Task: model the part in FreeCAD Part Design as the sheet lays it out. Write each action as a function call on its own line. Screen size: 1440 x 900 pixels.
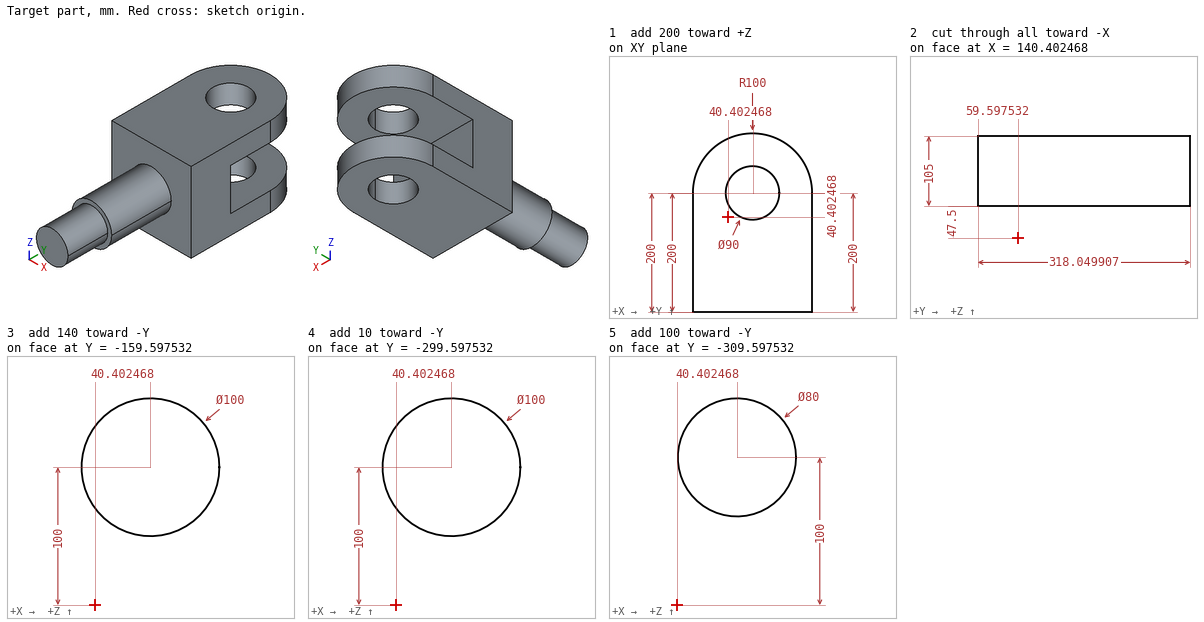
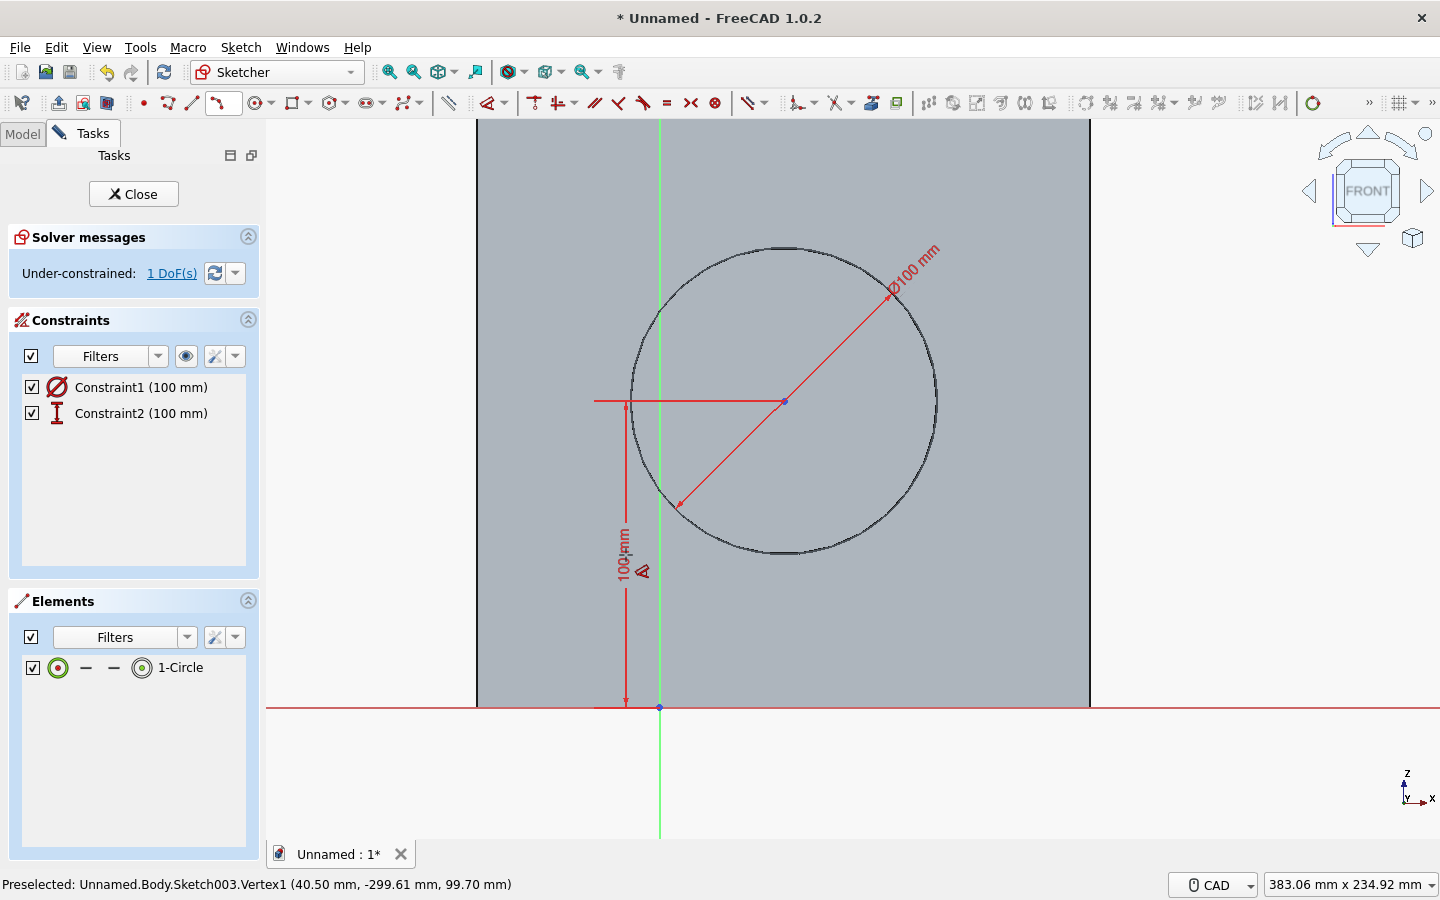
click(784, 401)
click(722, 742)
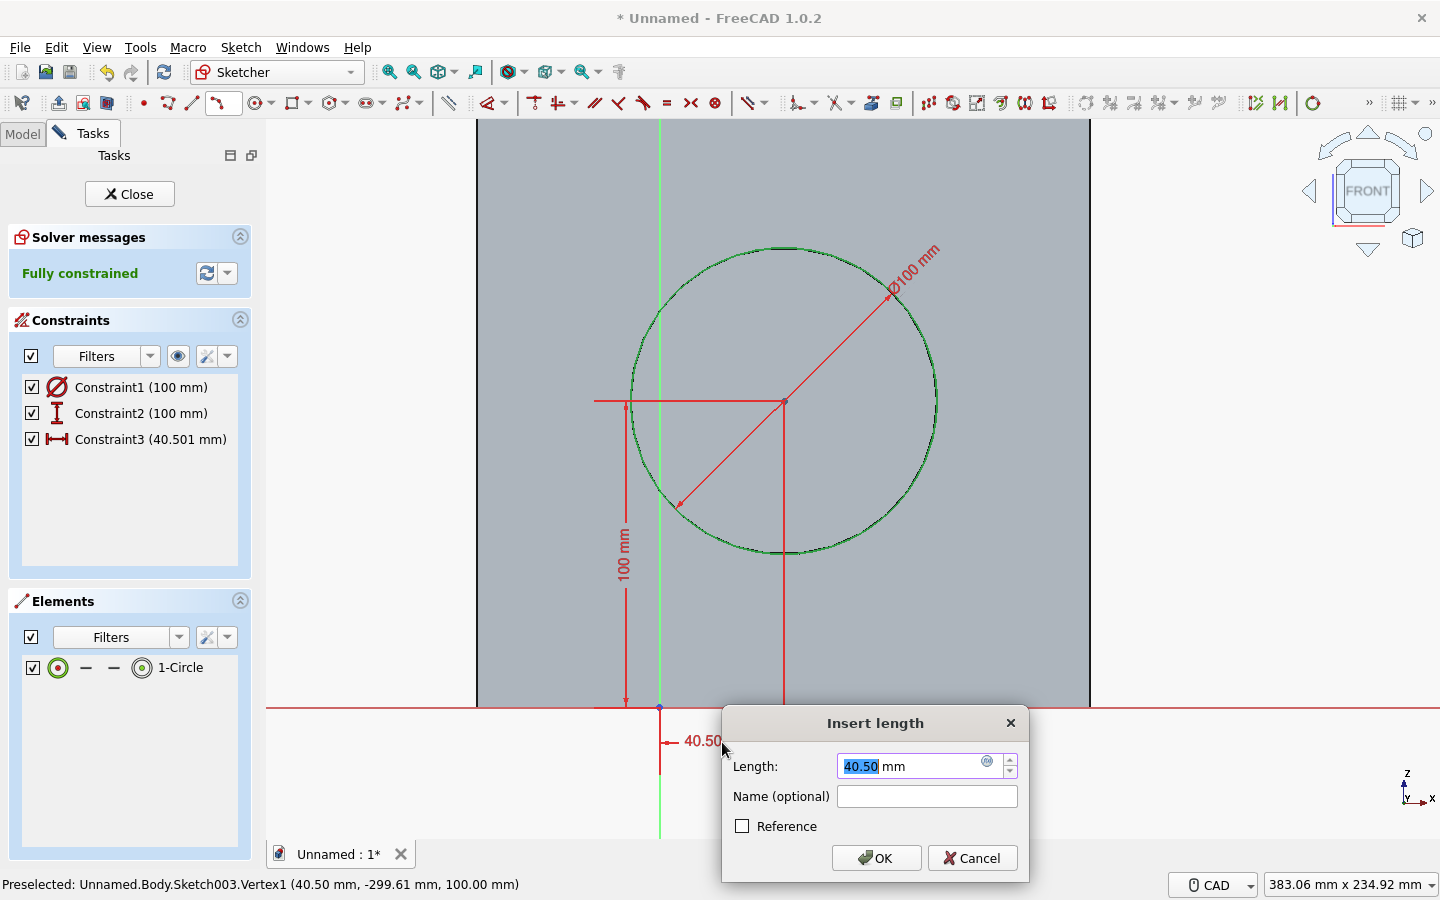
text(40.402468)
key(Return)
key(Escape)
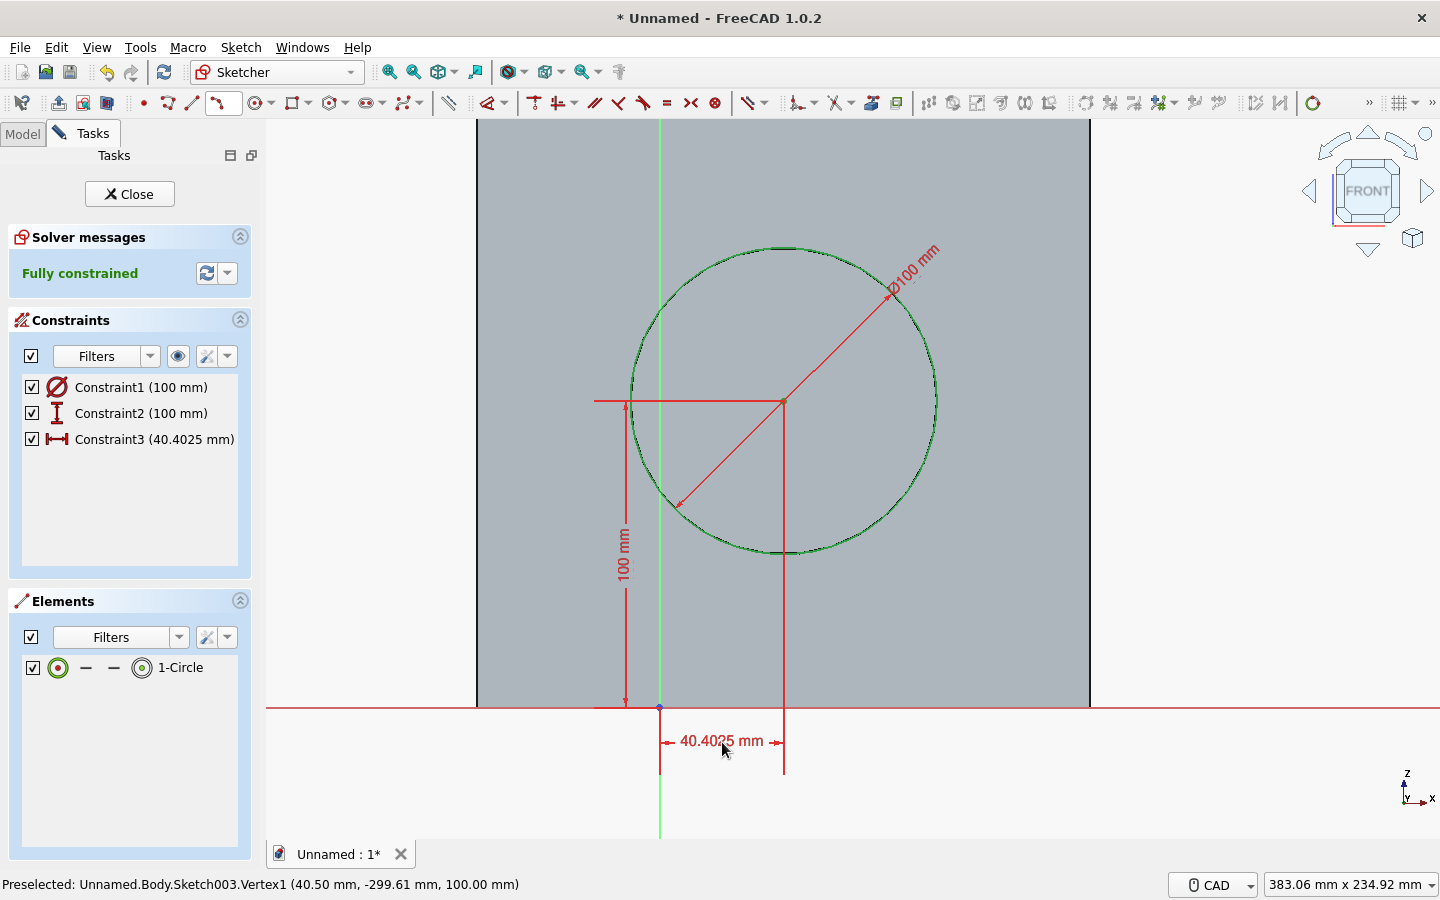
click(130, 194)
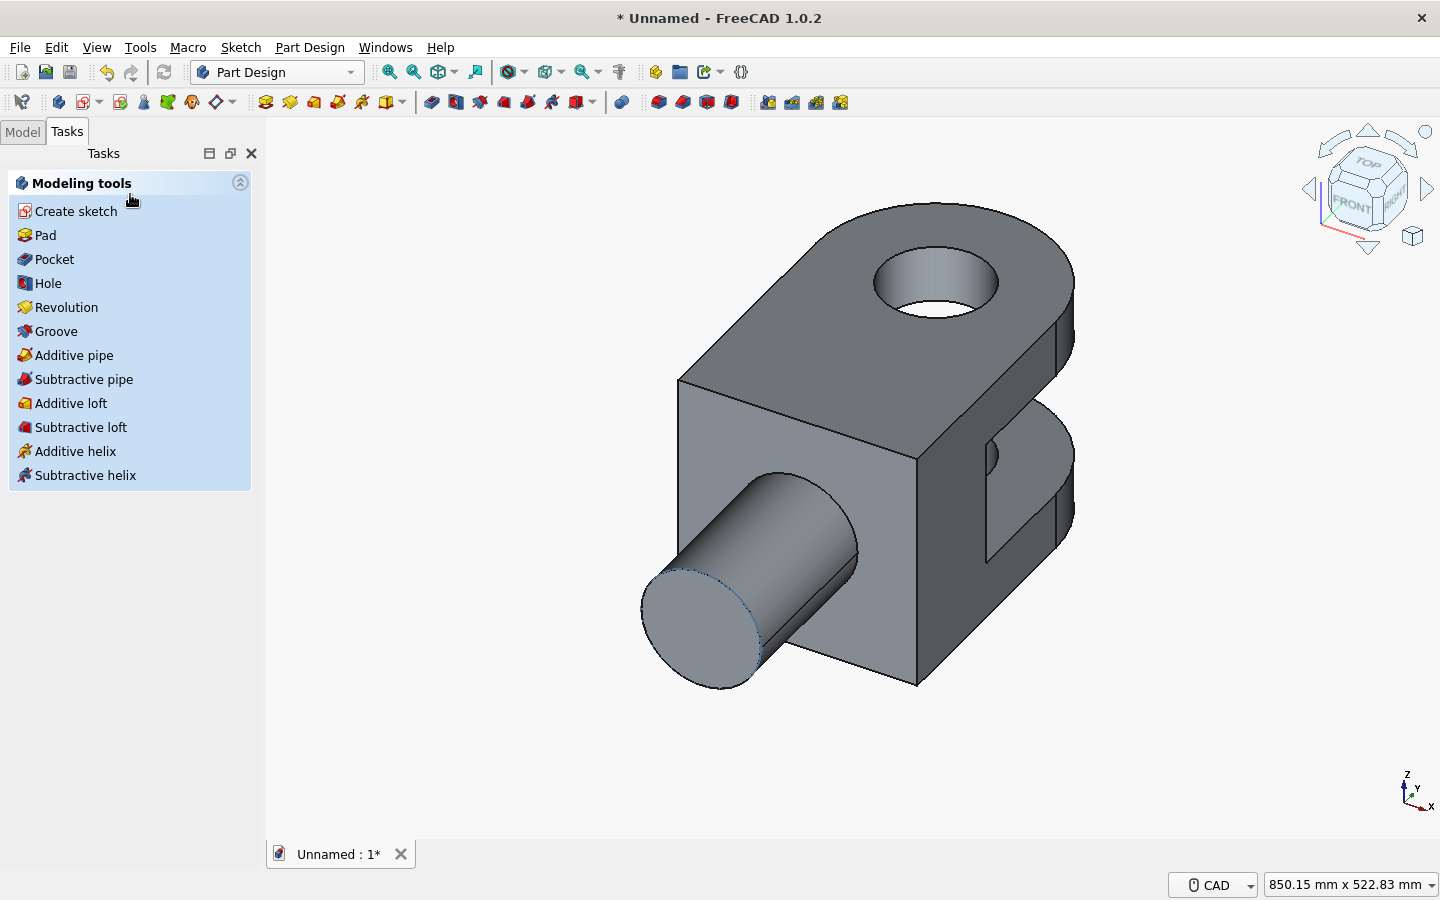
click(266, 102)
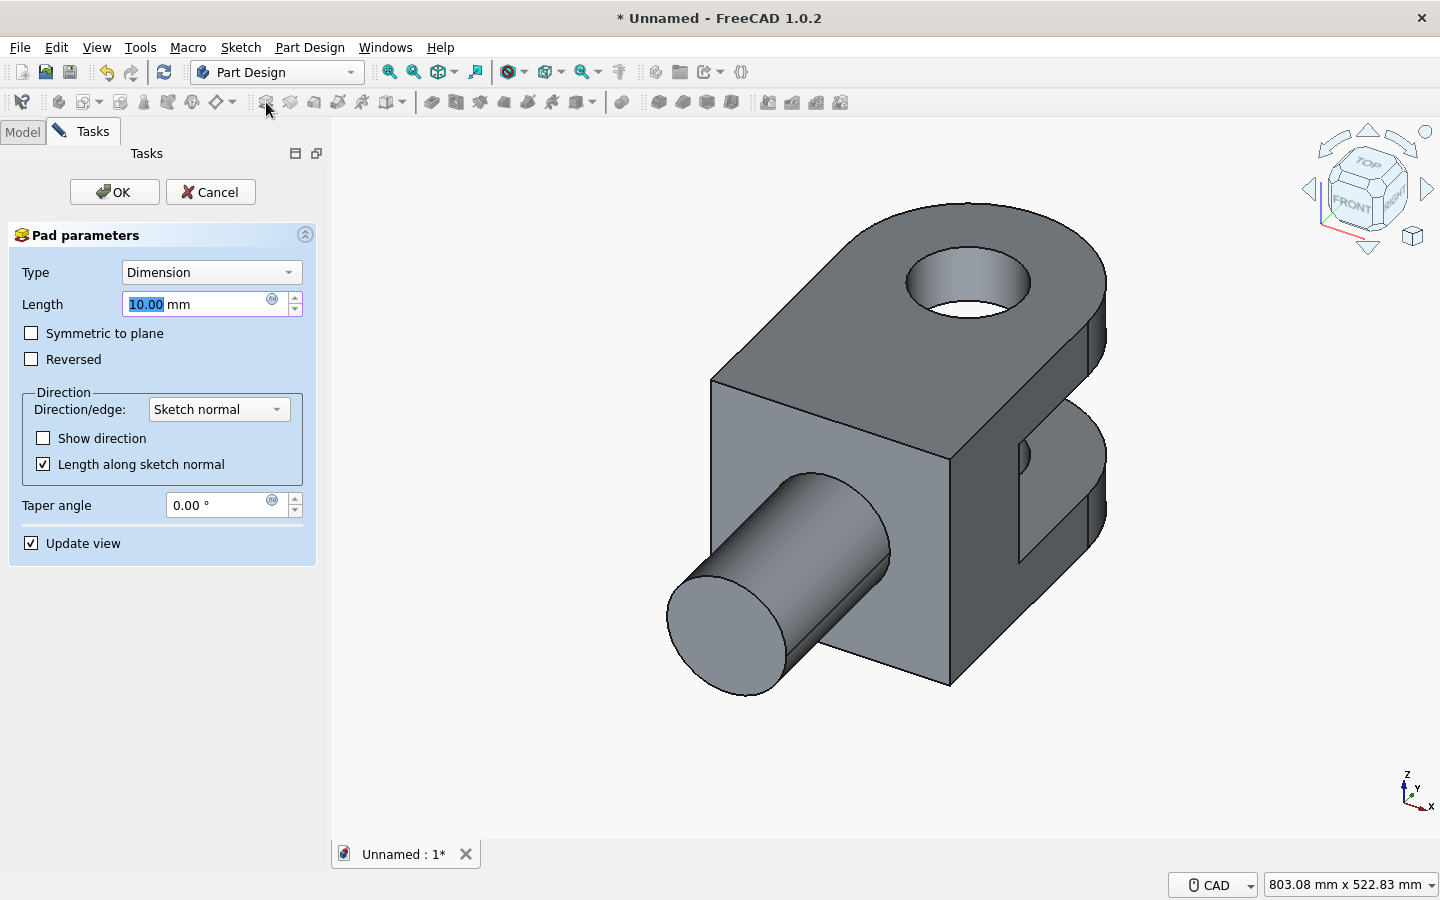
text(10)
key(Tab)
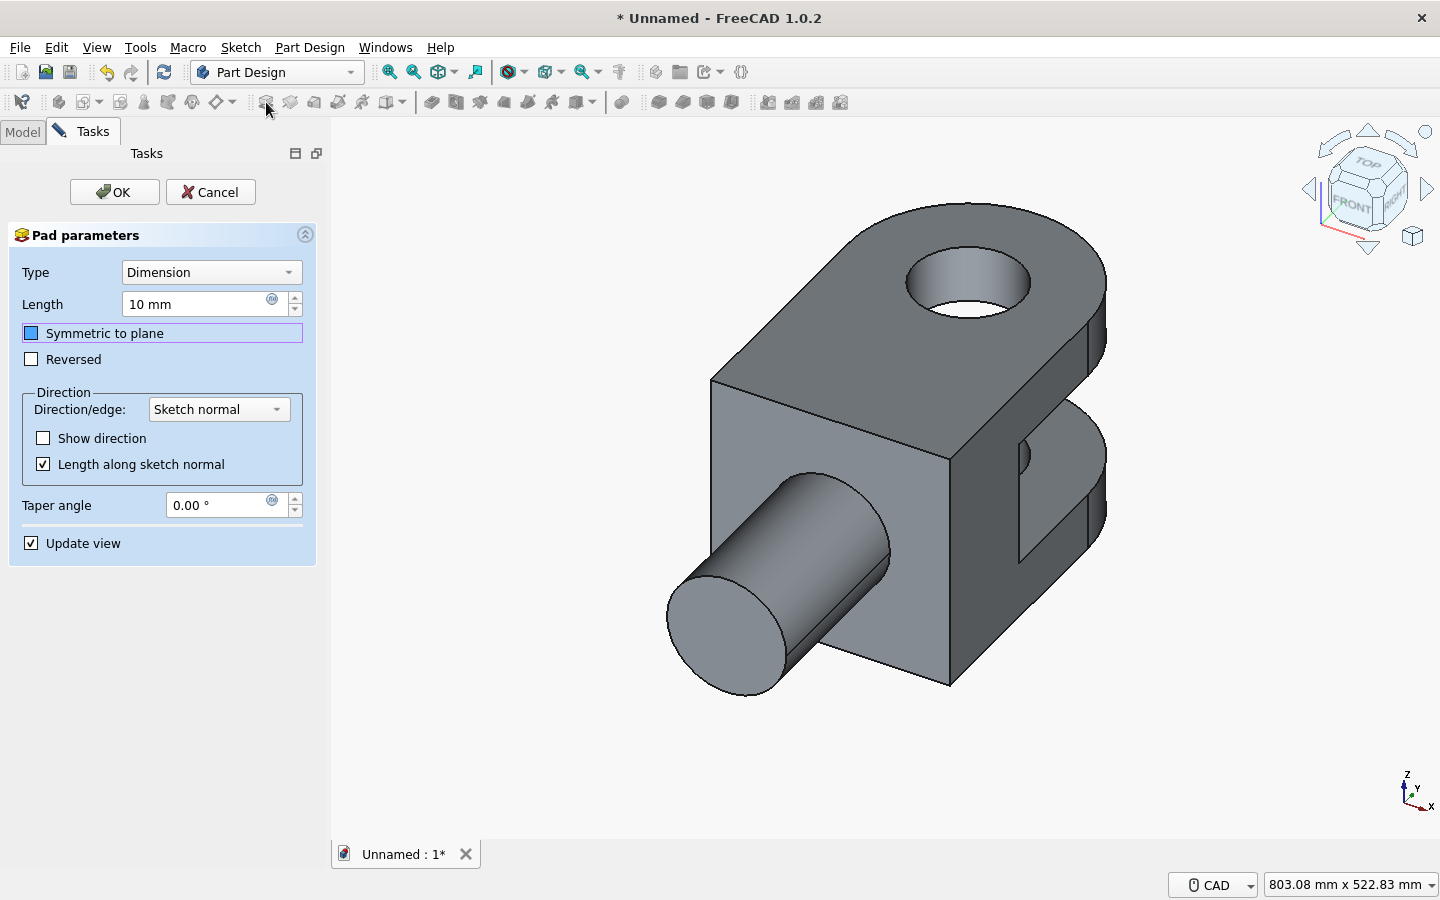
click(115, 192)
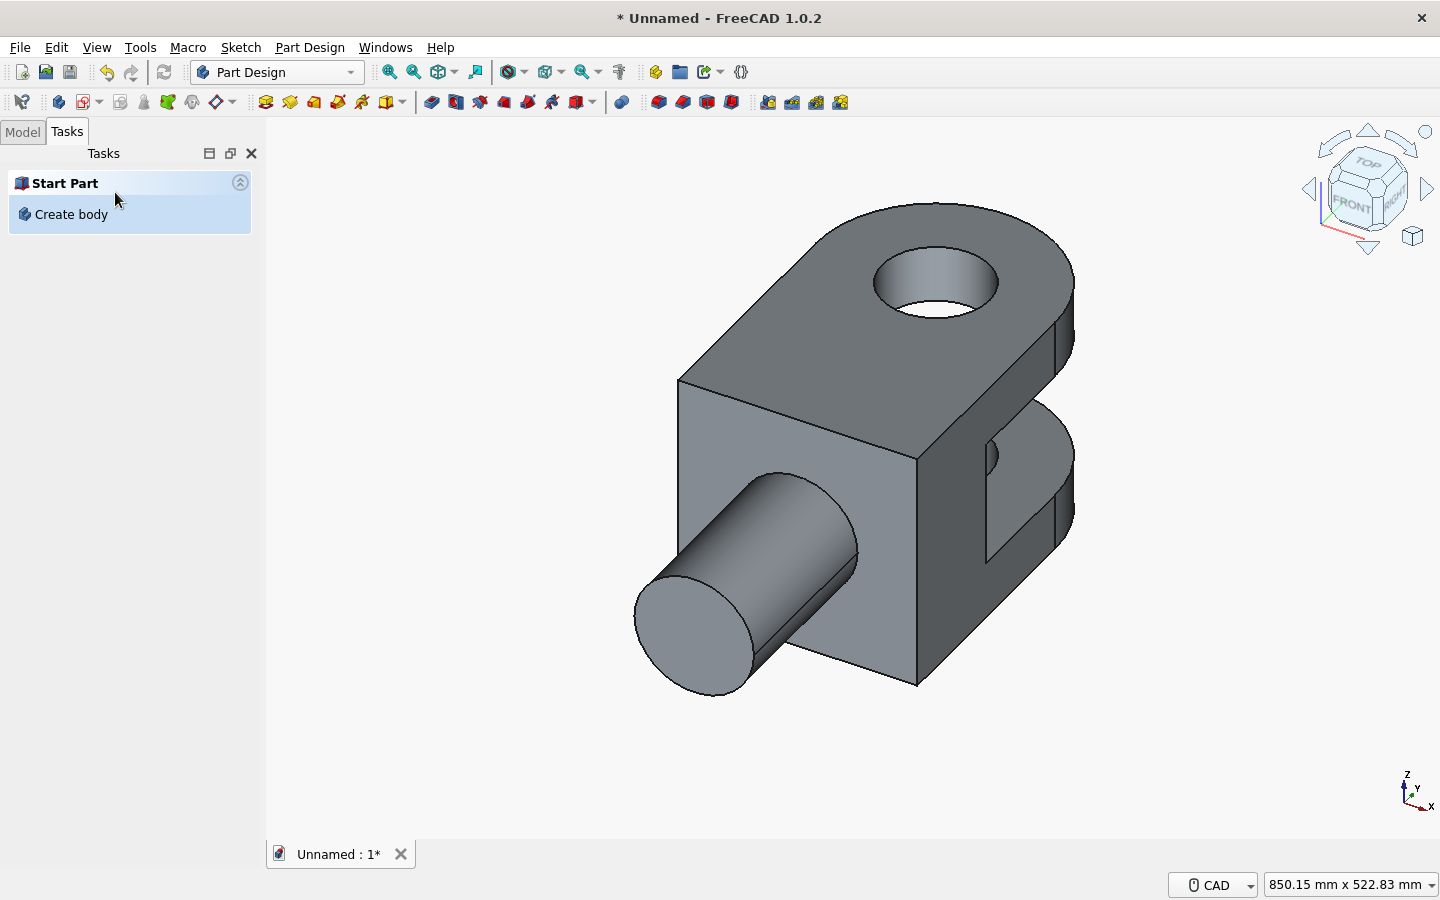
click(694, 635)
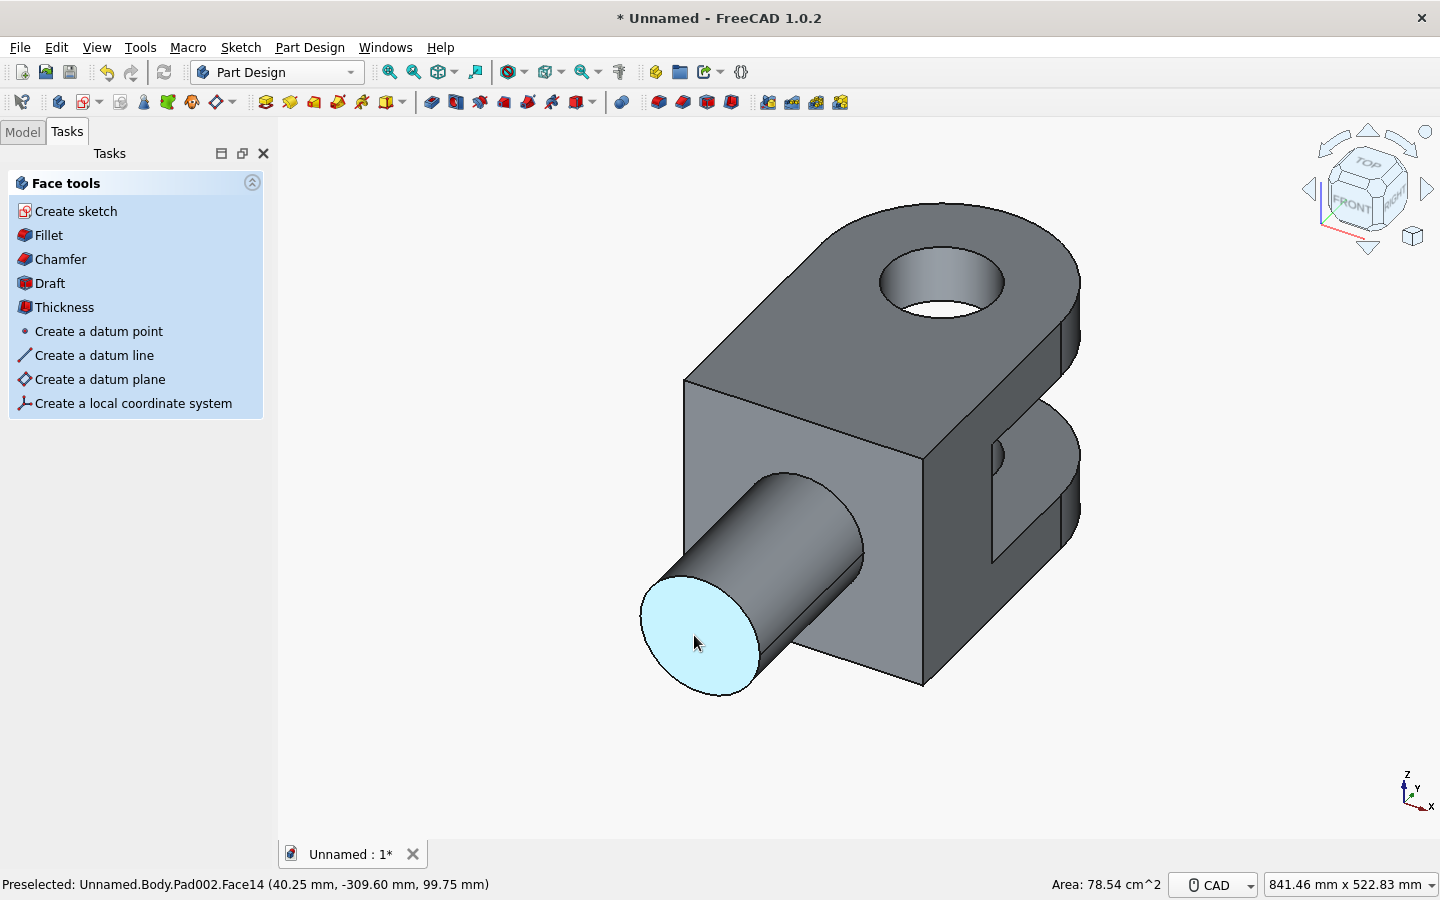
click(84, 102)